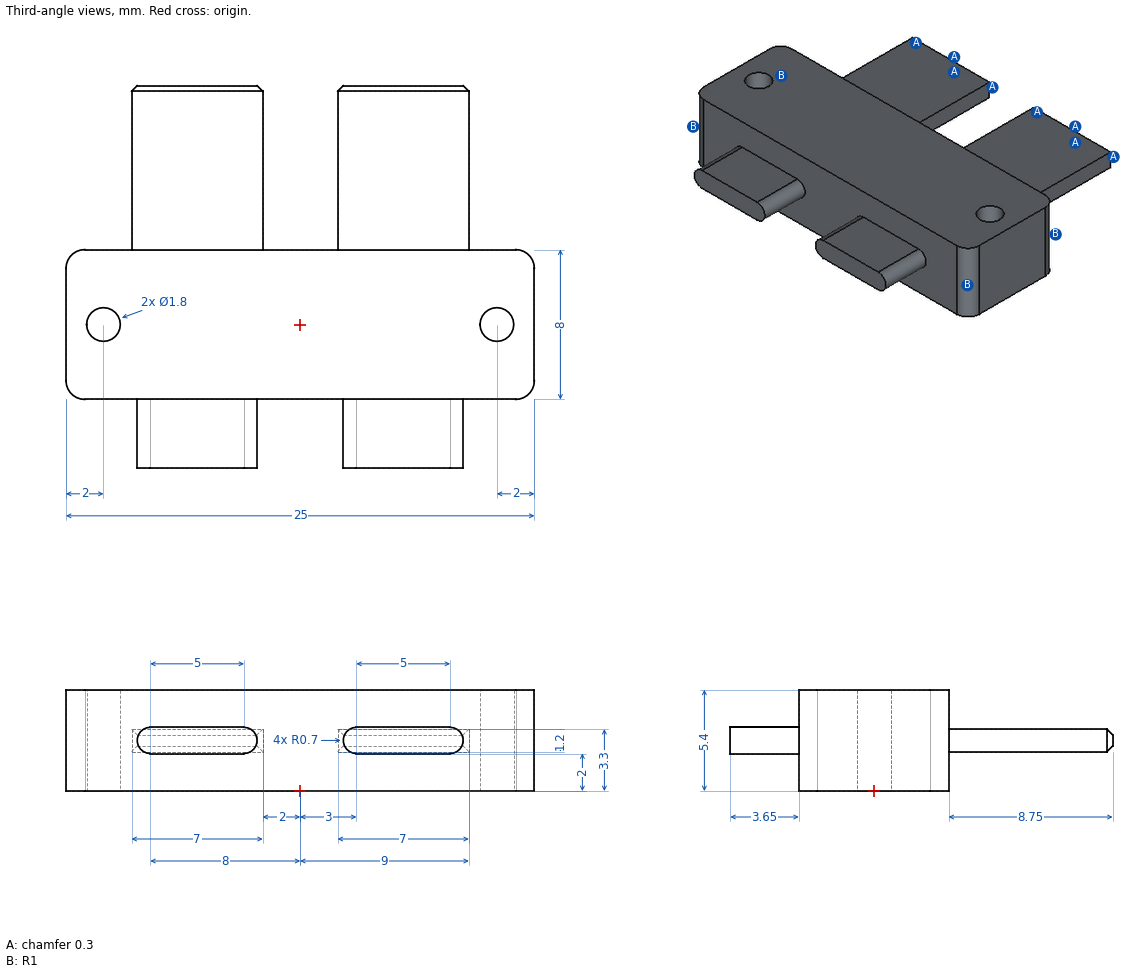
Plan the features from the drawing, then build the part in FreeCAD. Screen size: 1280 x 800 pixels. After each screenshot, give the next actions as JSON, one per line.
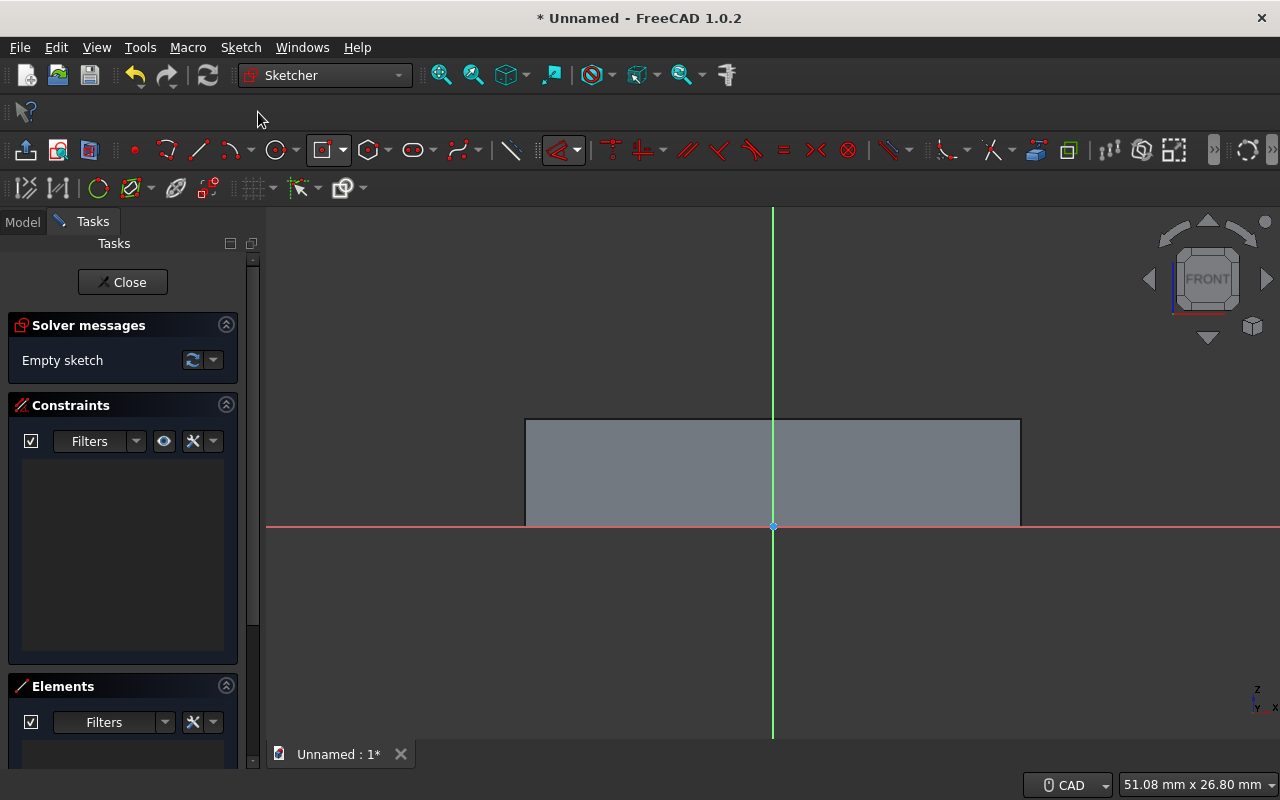
{"action": "scroll", "coordinate": [856, 517], "scroll_direction": "up", "scroll_amount": 3}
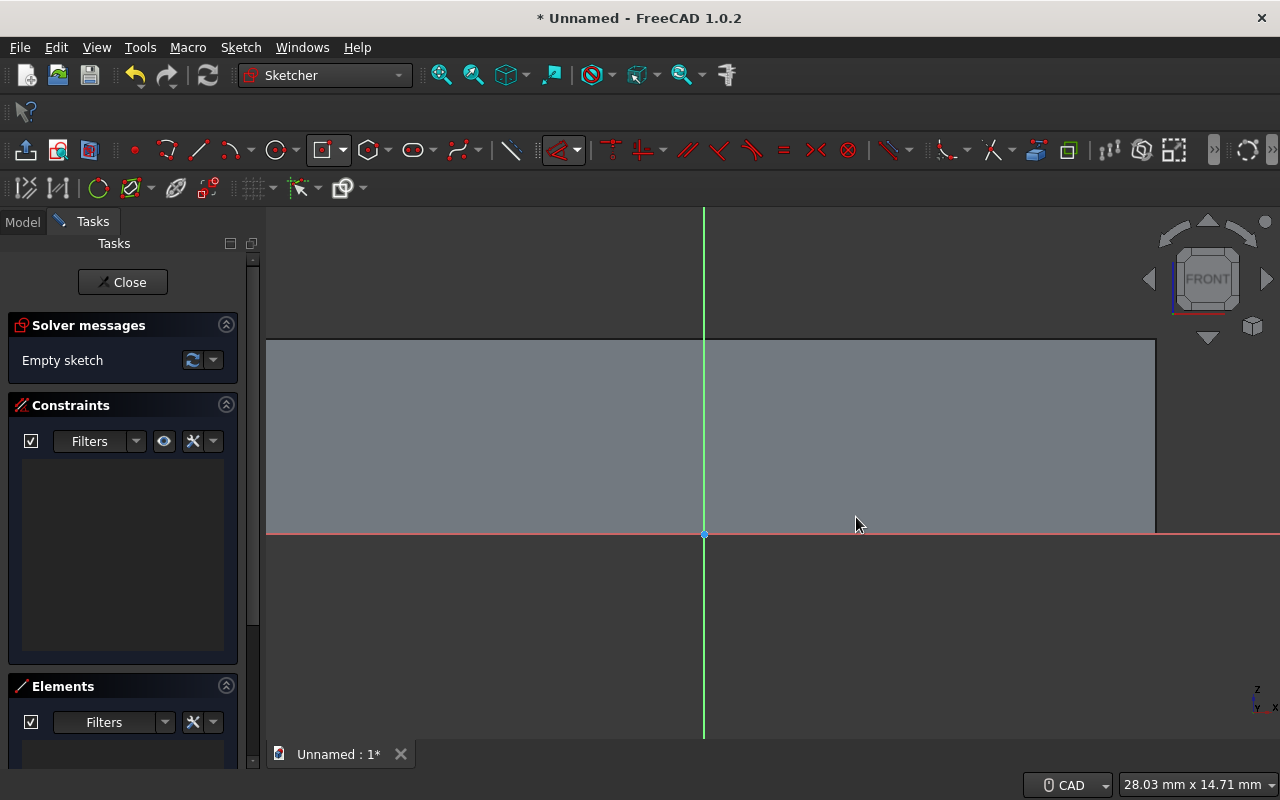
{"action": "left_click", "coordinate": [414, 150]}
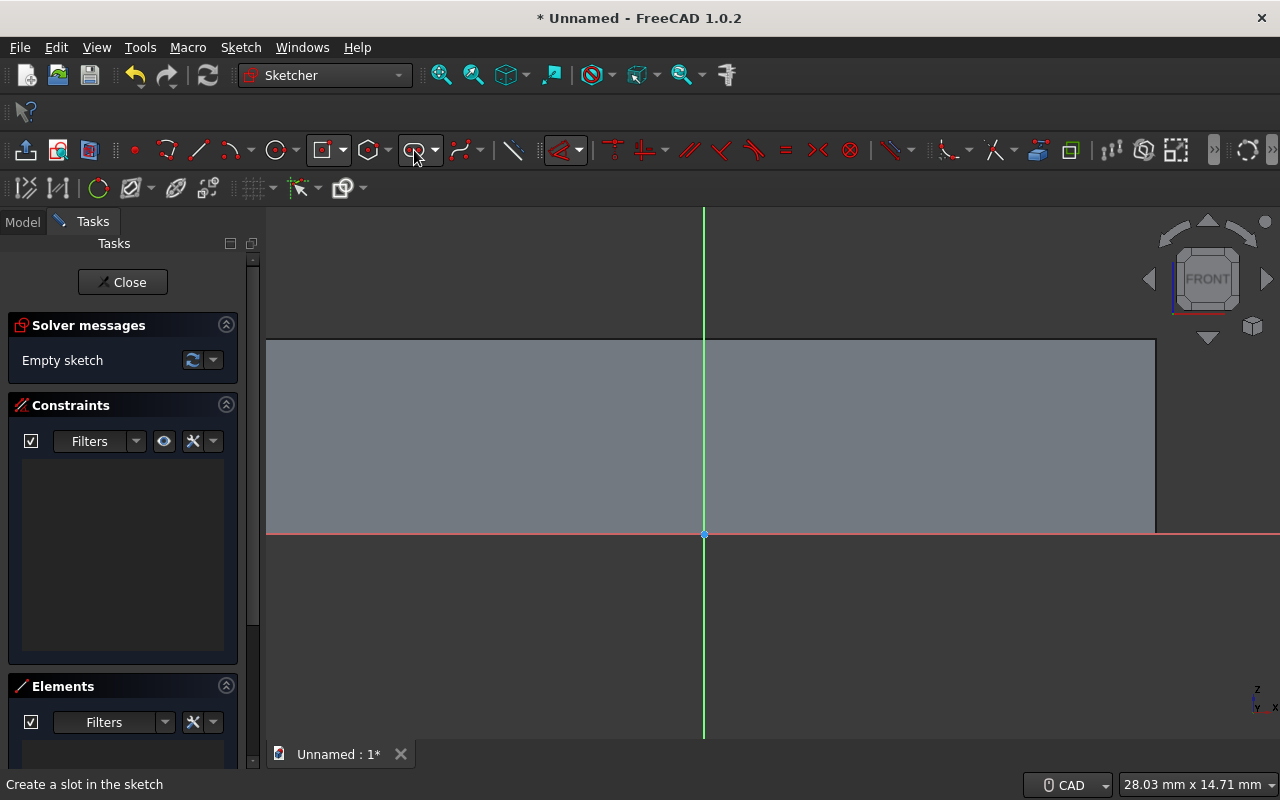
{"action": "left_click", "coordinate": [813, 436]}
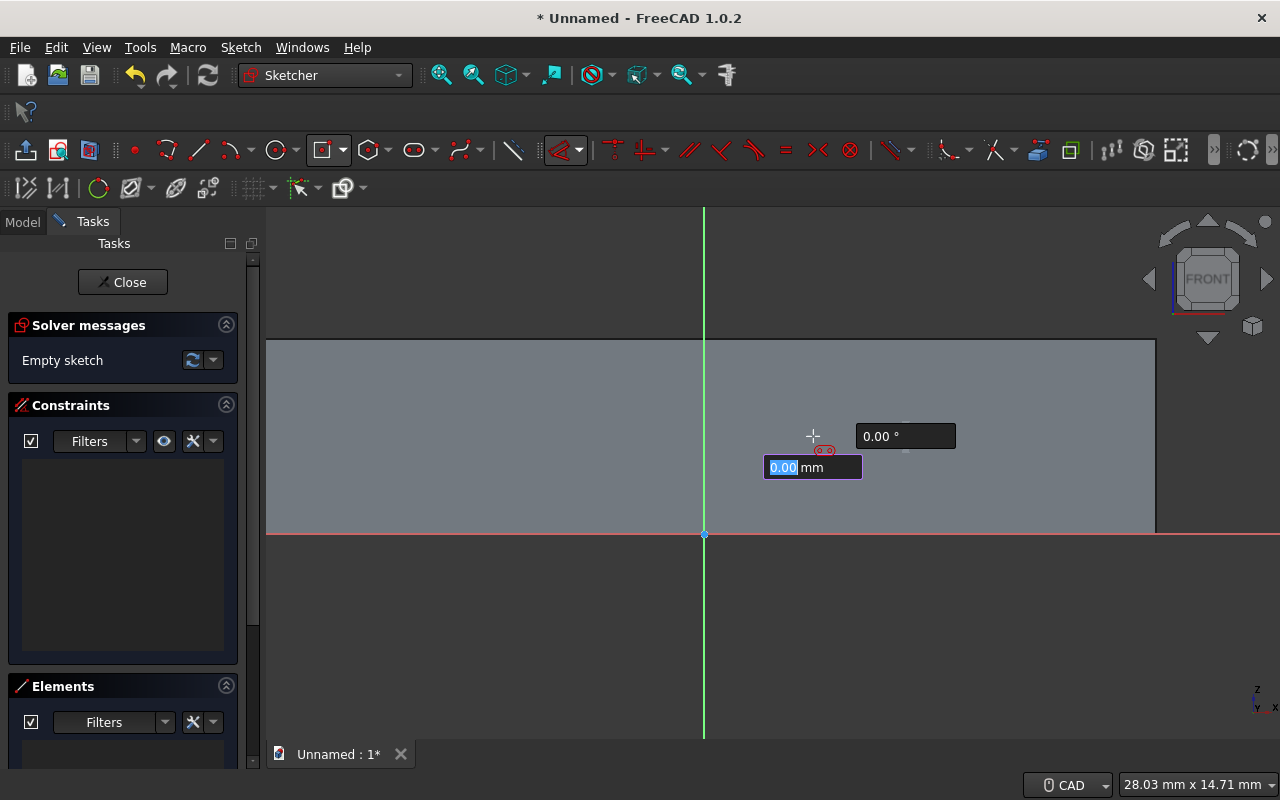
{"action": "left_click", "coordinate": [994, 436]}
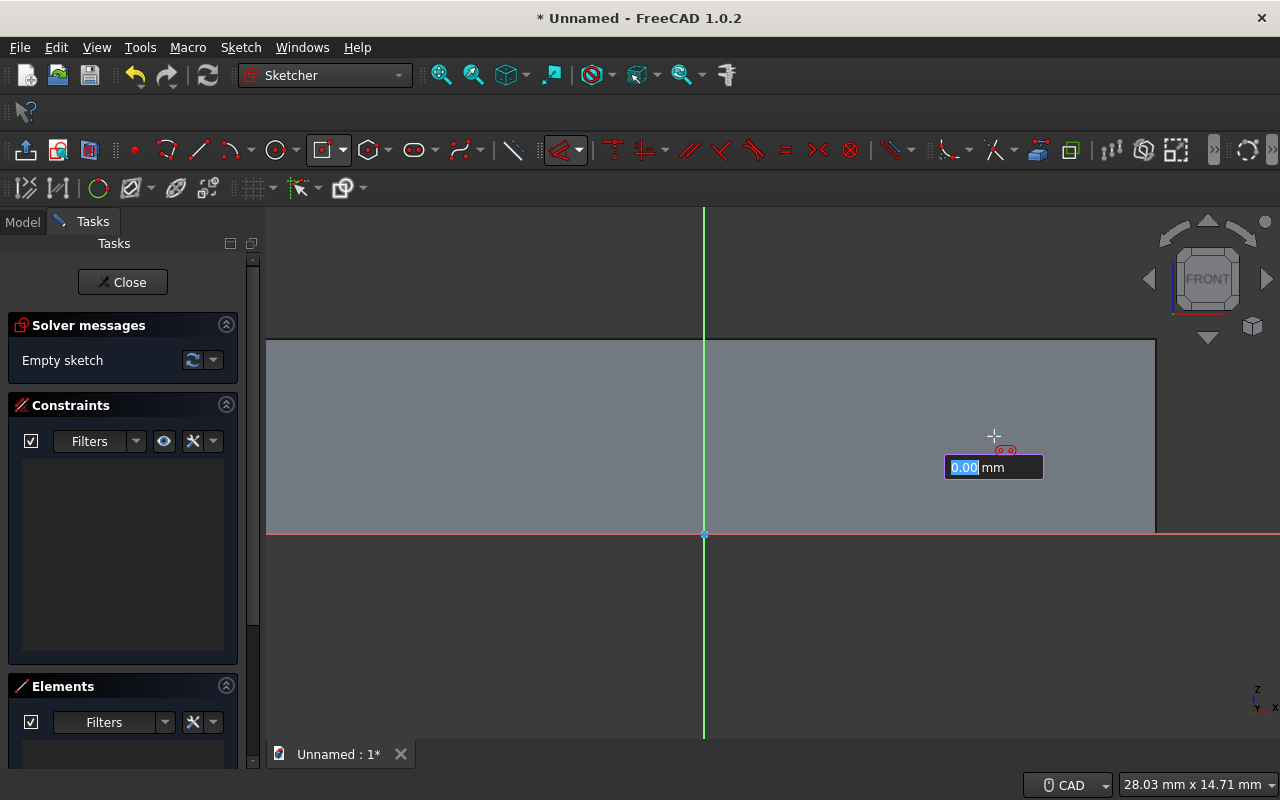
{"action": "left_click", "coordinate": [903, 411]}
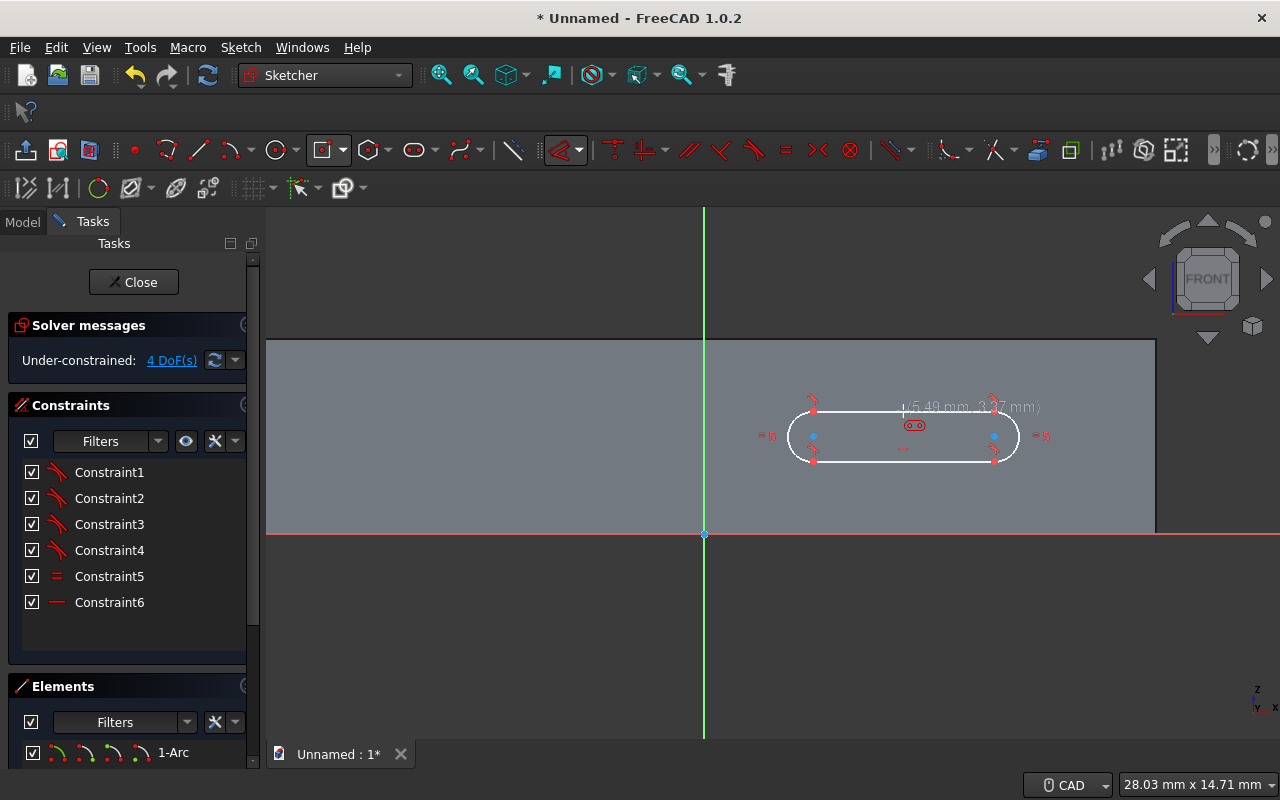
{"action": "left_click", "coordinate": [415, 436]}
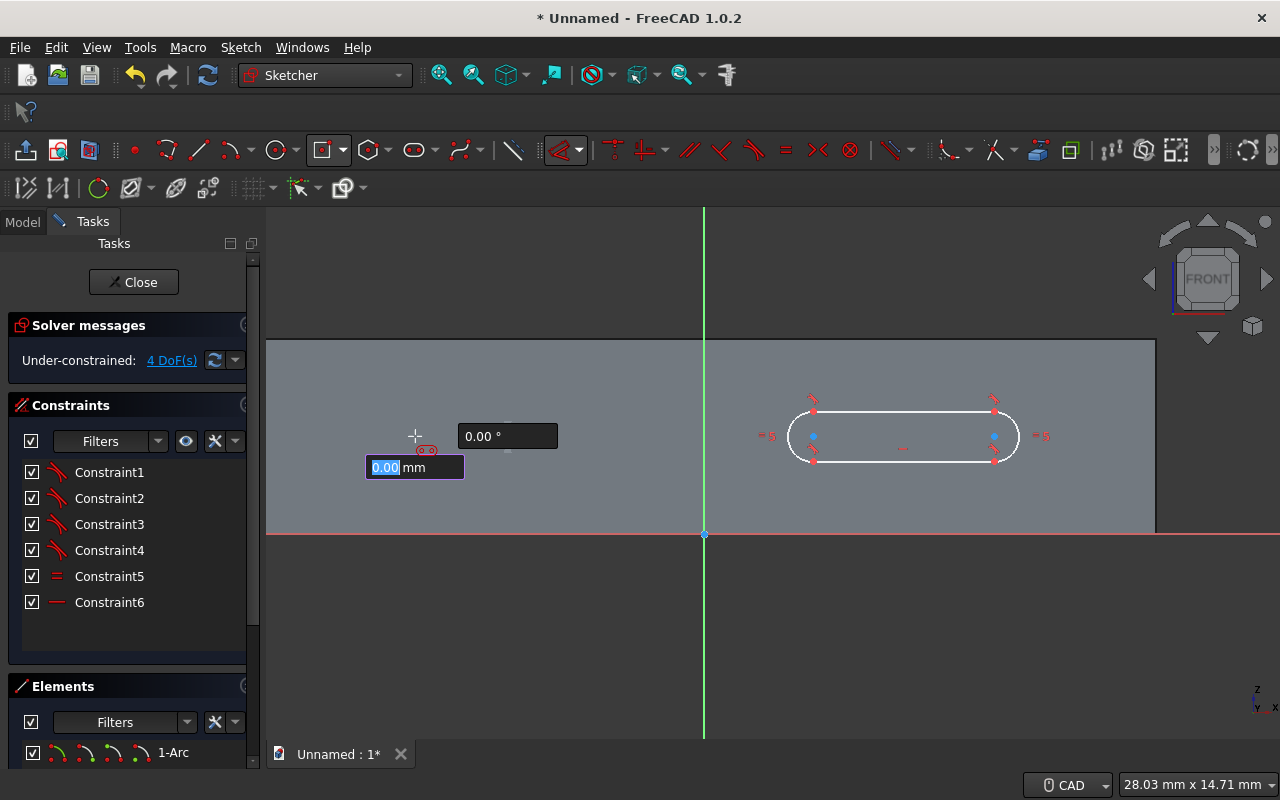
{"action": "left_click", "coordinate": [596, 436]}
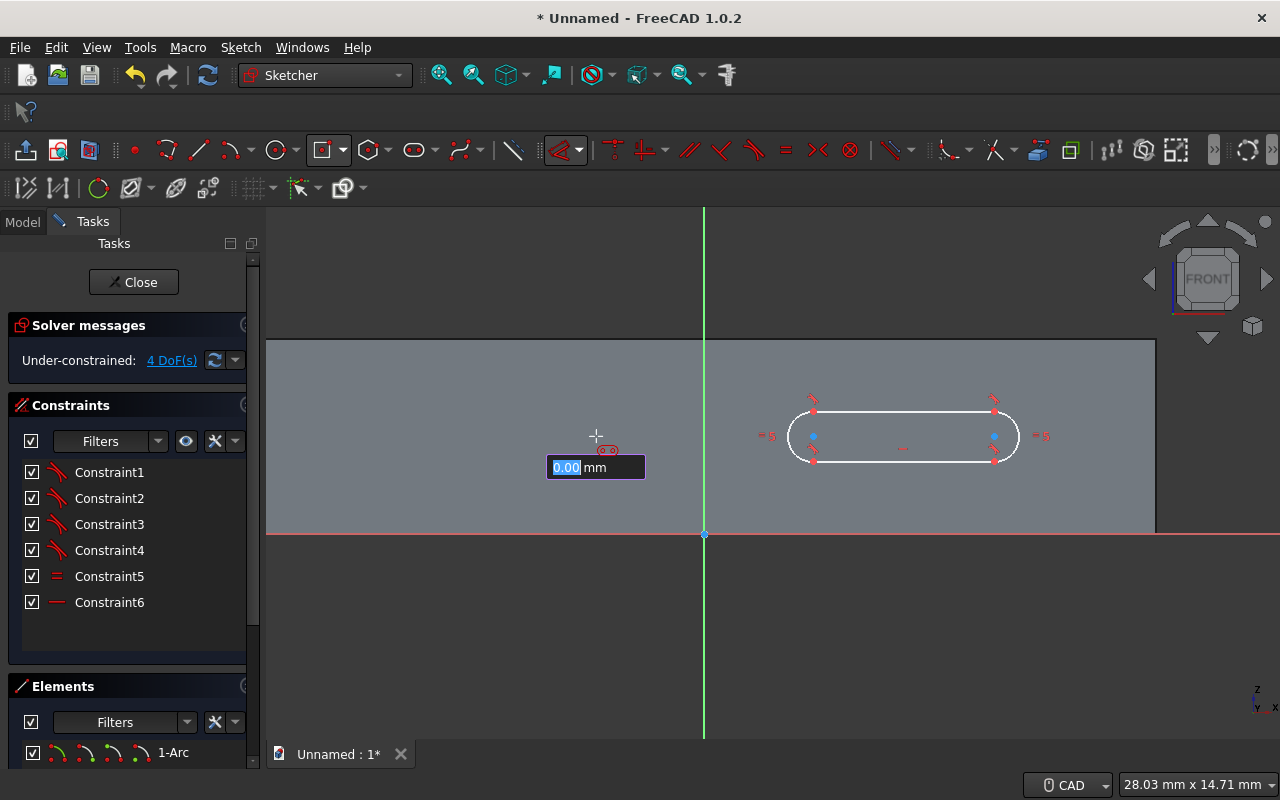
{"action": "left_click", "coordinate": [505, 411]}
{"action": "key", "text": "Escape"}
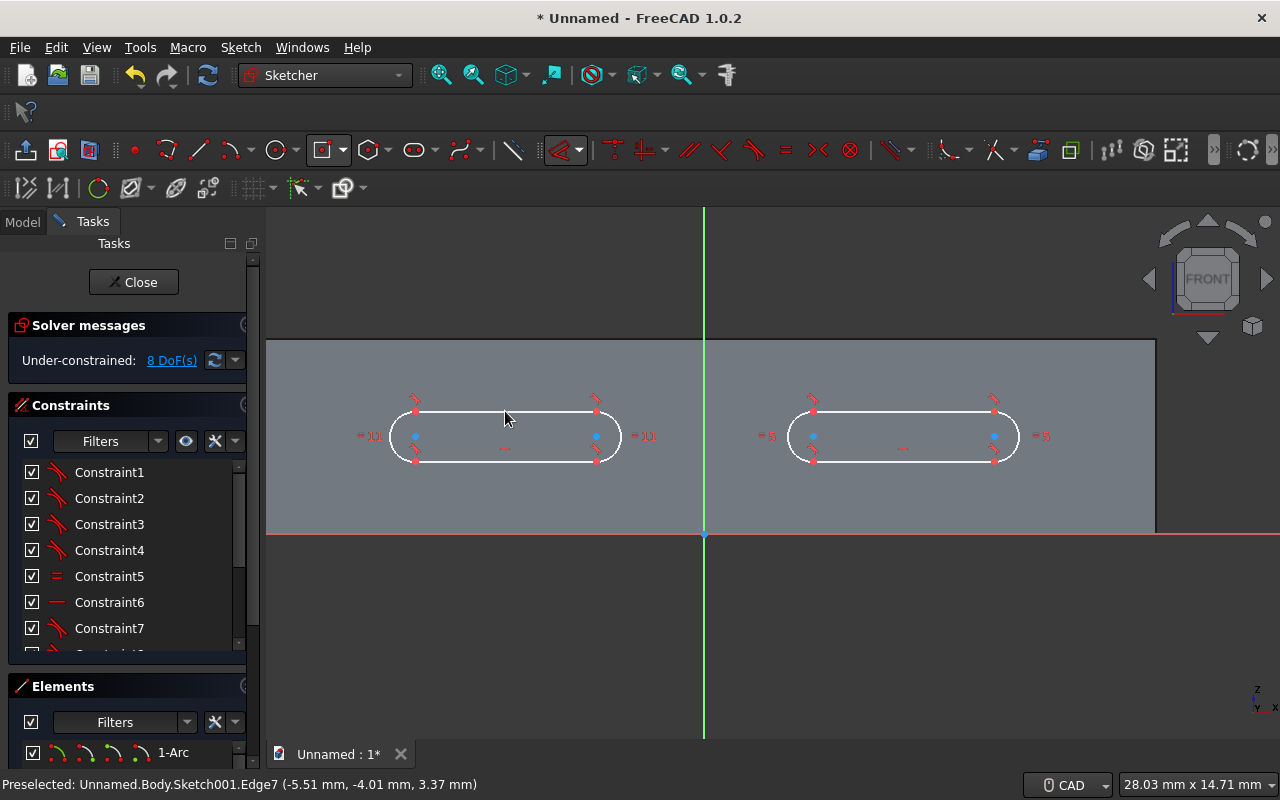
{"action": "left_click", "coordinate": [793, 422]}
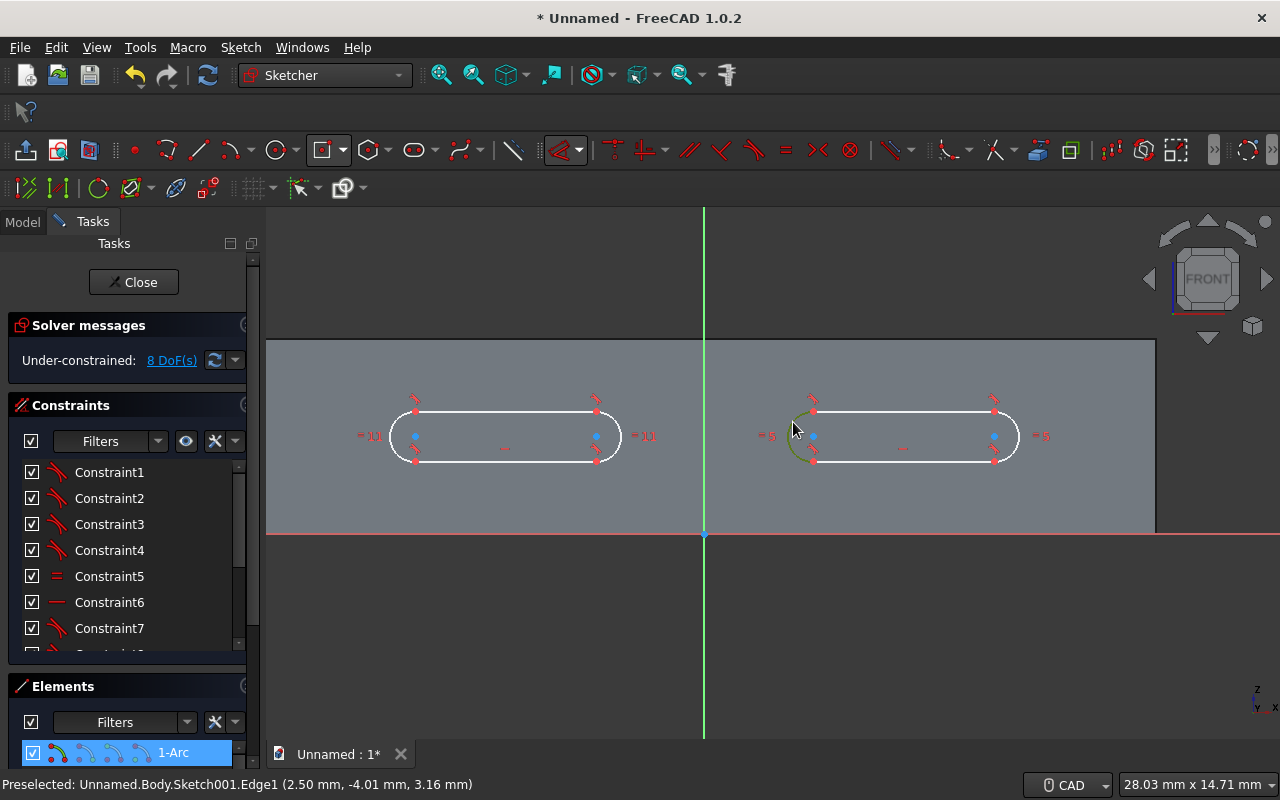
{"action": "left_click", "coordinate": [395, 422]}